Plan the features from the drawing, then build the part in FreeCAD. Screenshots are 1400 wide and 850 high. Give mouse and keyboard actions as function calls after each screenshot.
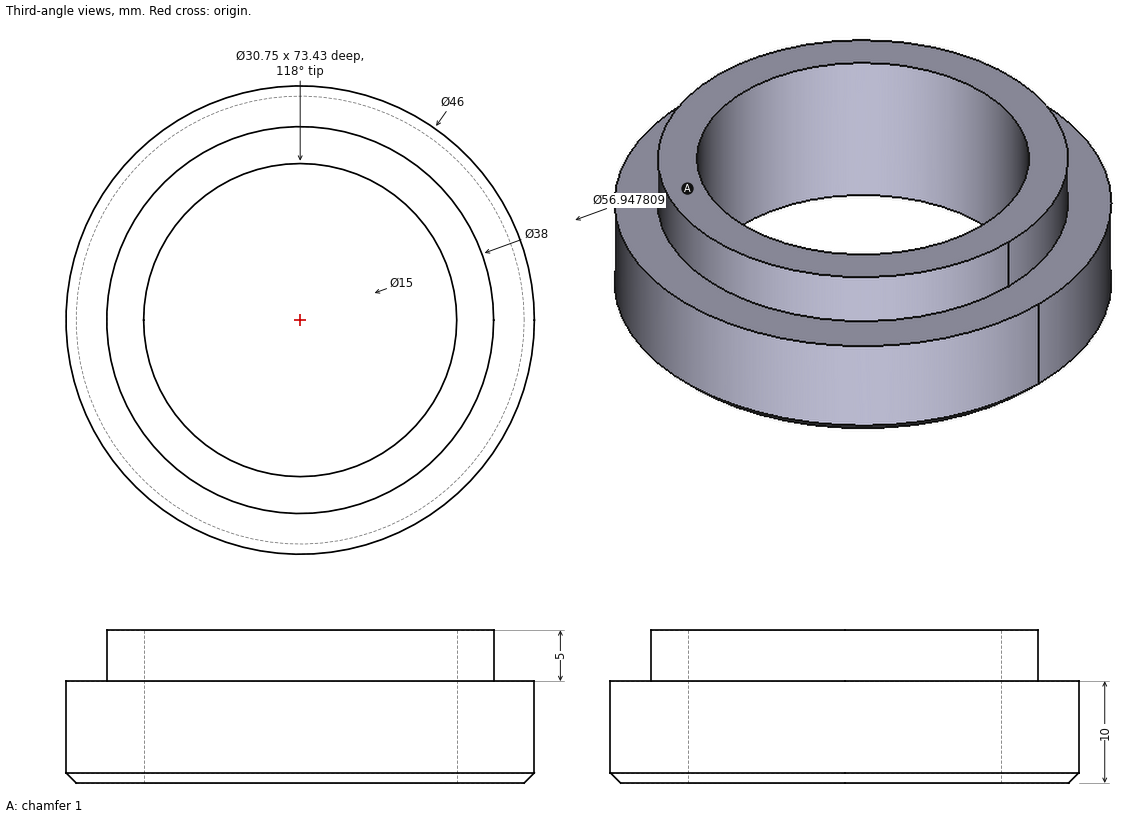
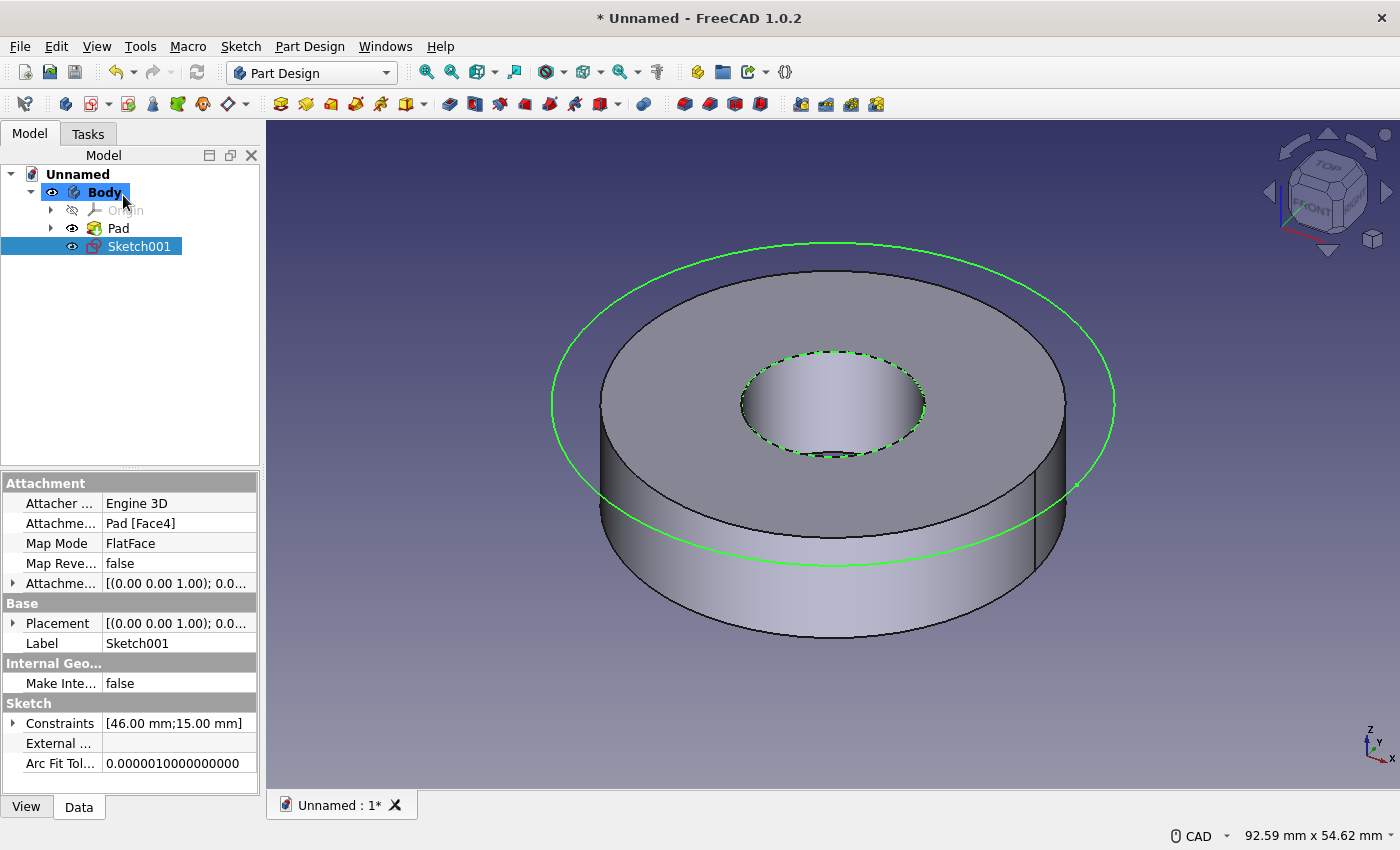
click(281, 104)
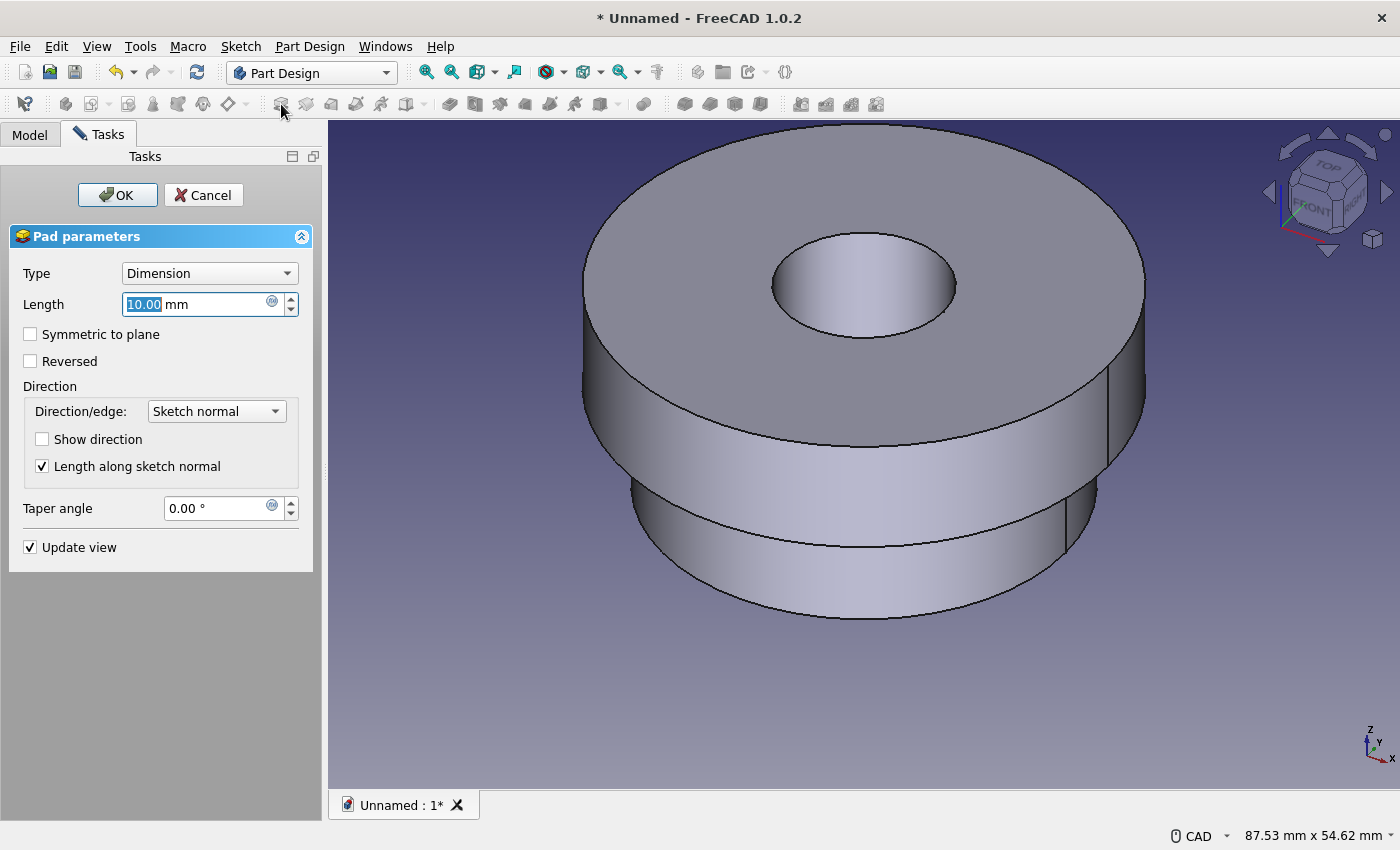
text(10)
key(Tab)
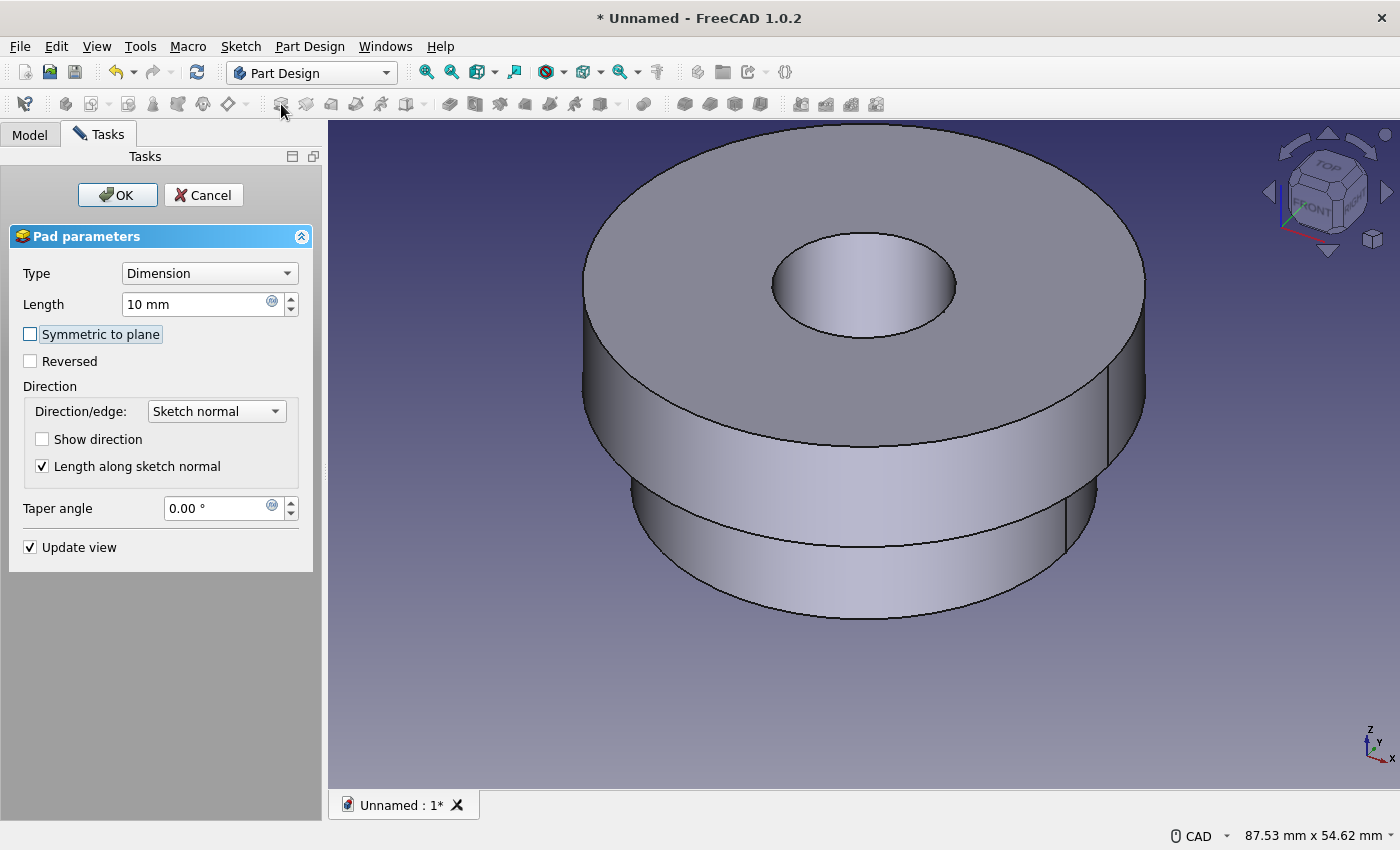
click(118, 195)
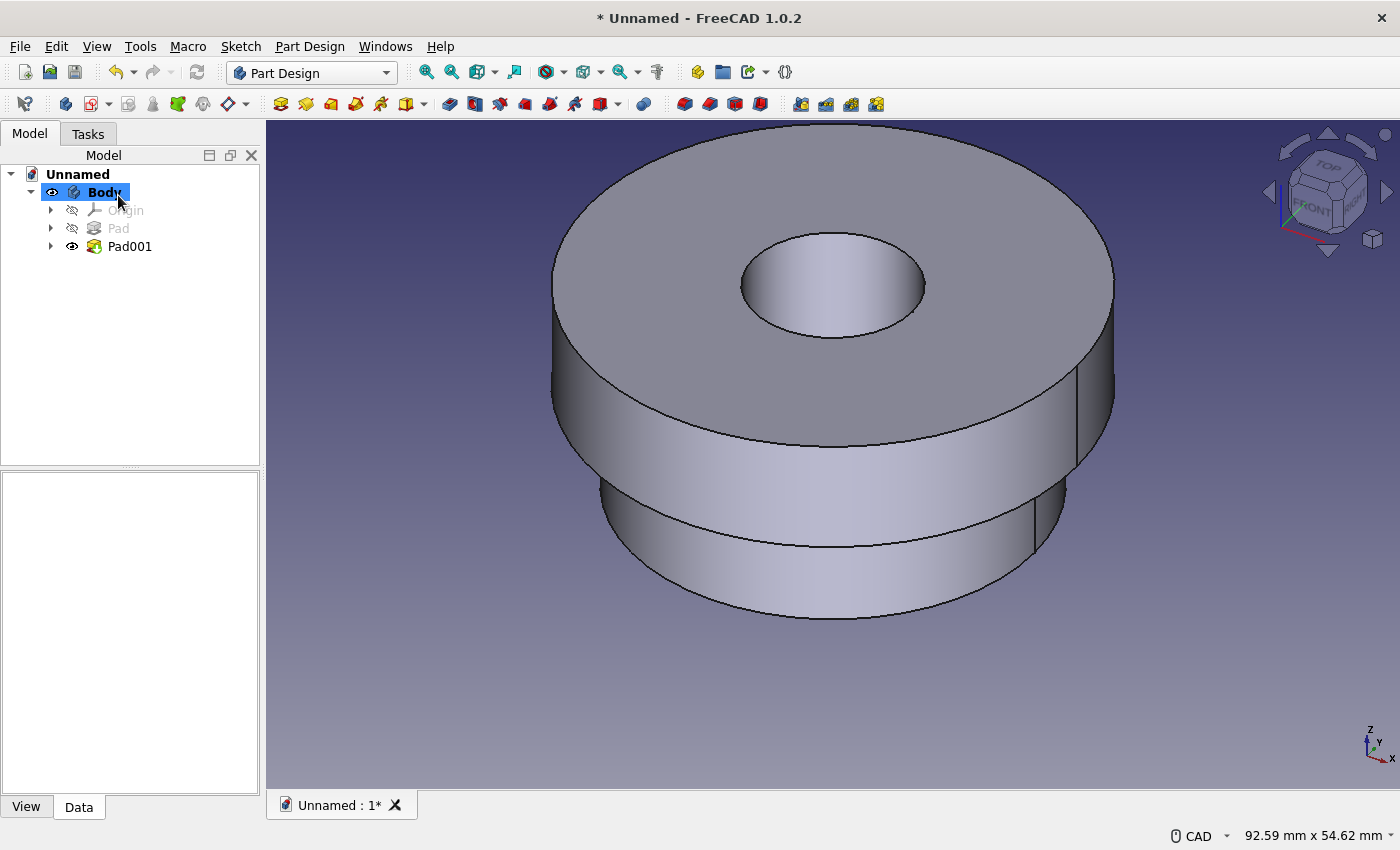
key(v)
key(f)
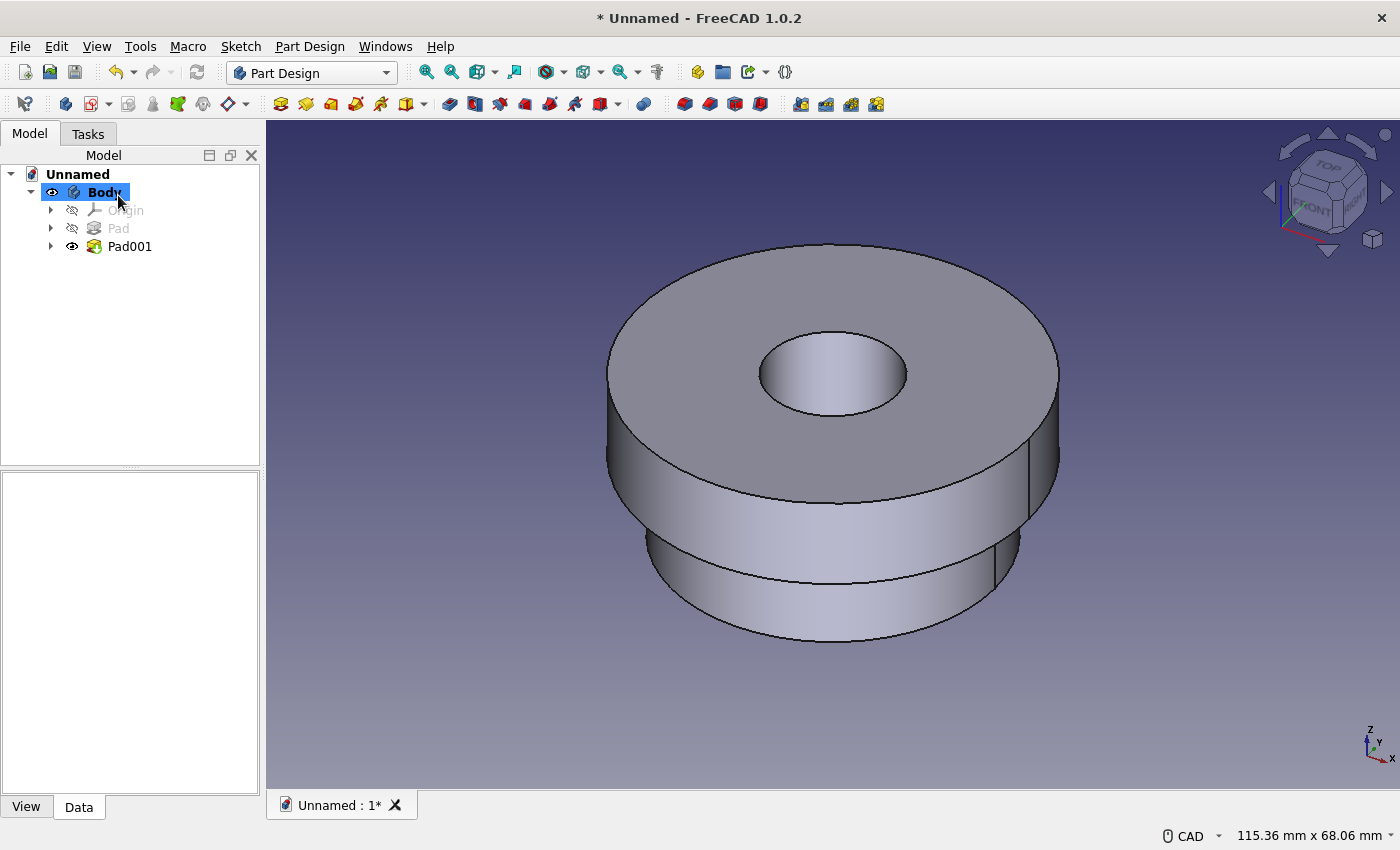
click(842, 290)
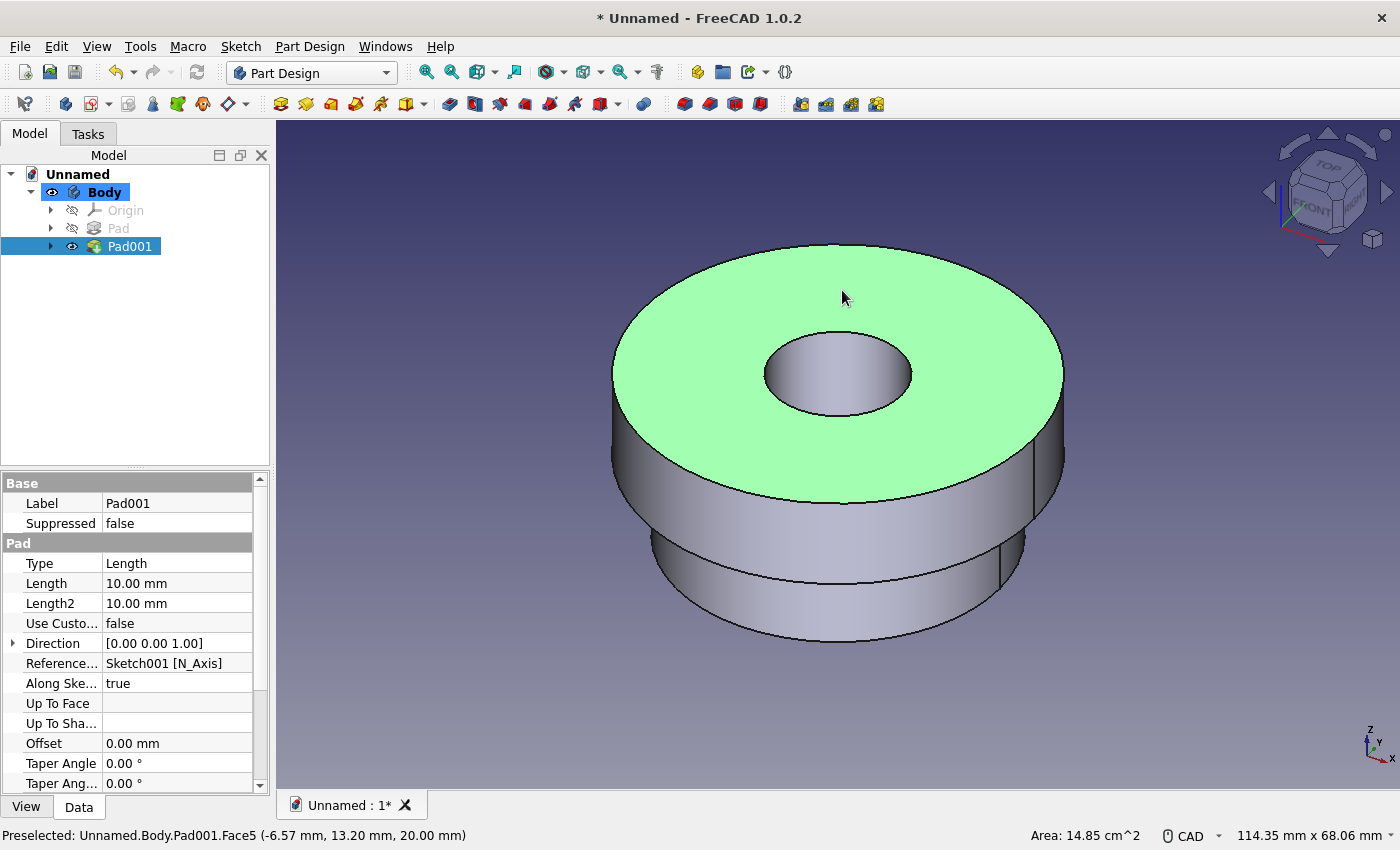
click(90, 104)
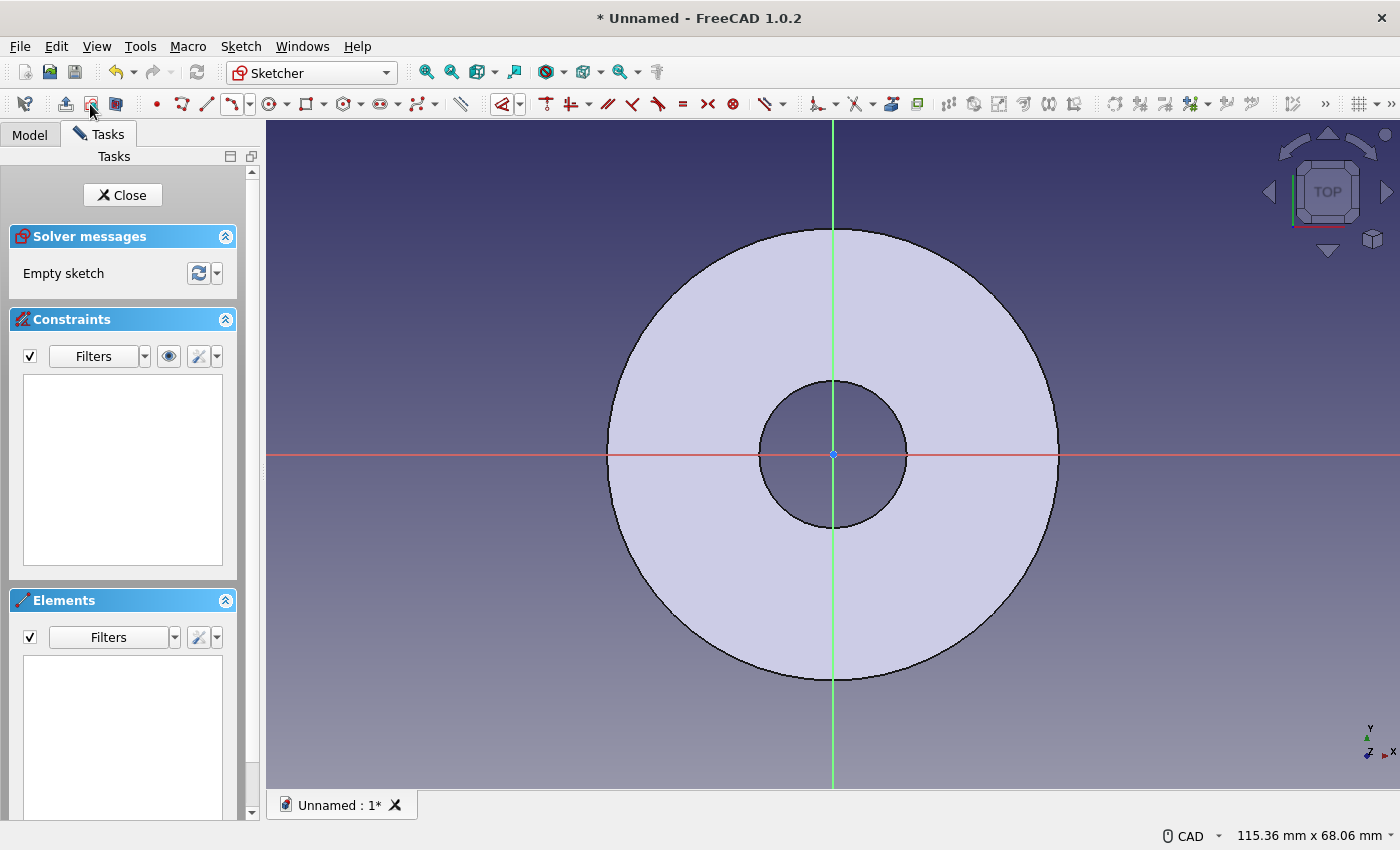
click(268, 104)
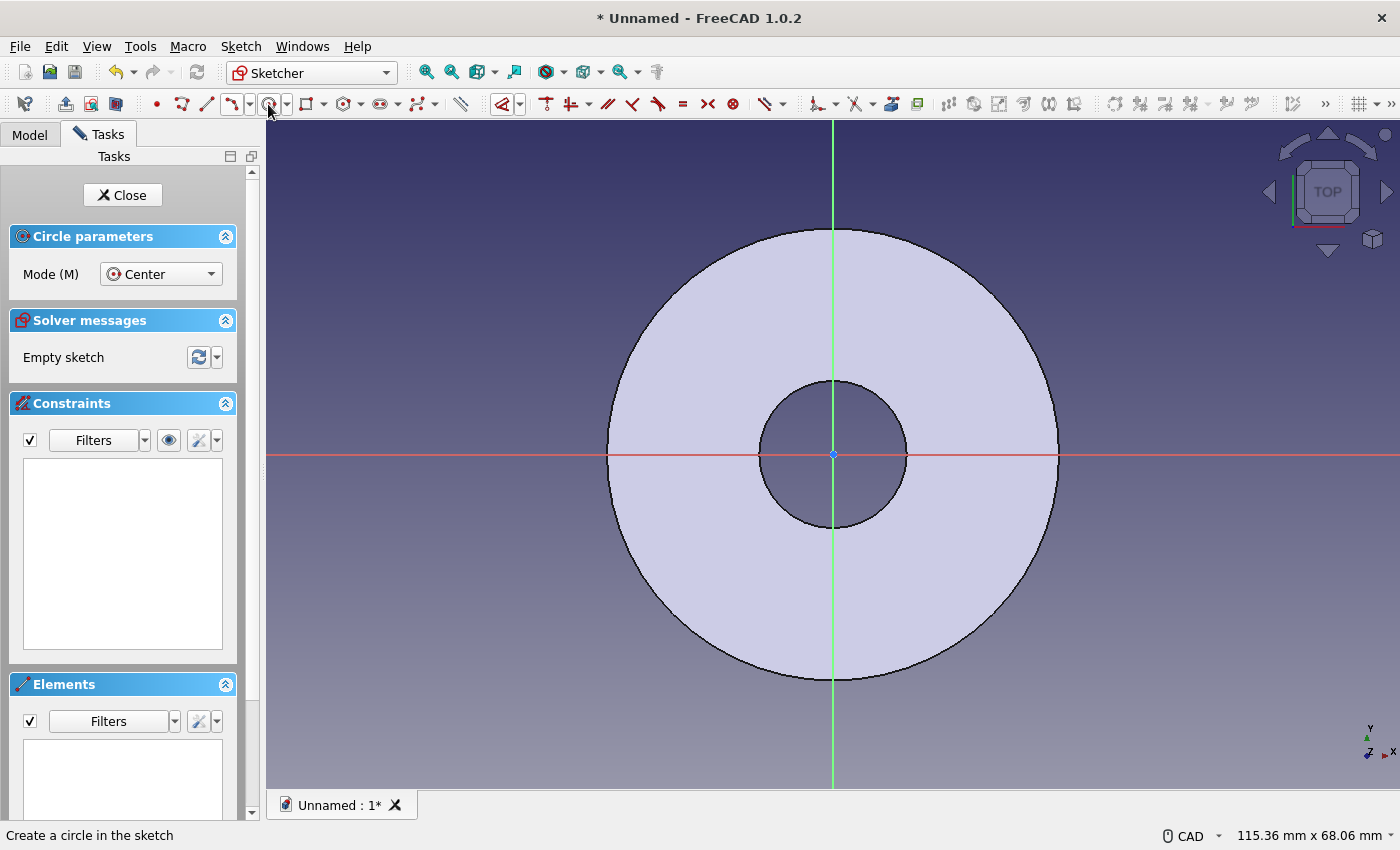
click(833, 454)
move(965, 322)